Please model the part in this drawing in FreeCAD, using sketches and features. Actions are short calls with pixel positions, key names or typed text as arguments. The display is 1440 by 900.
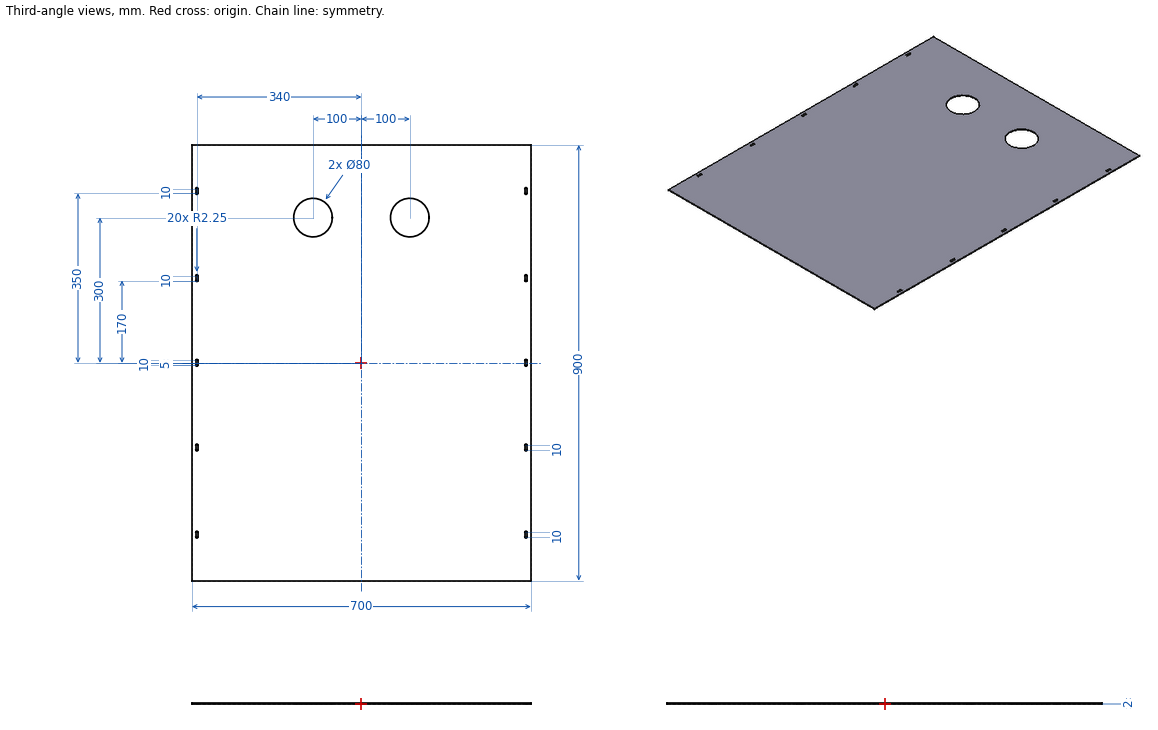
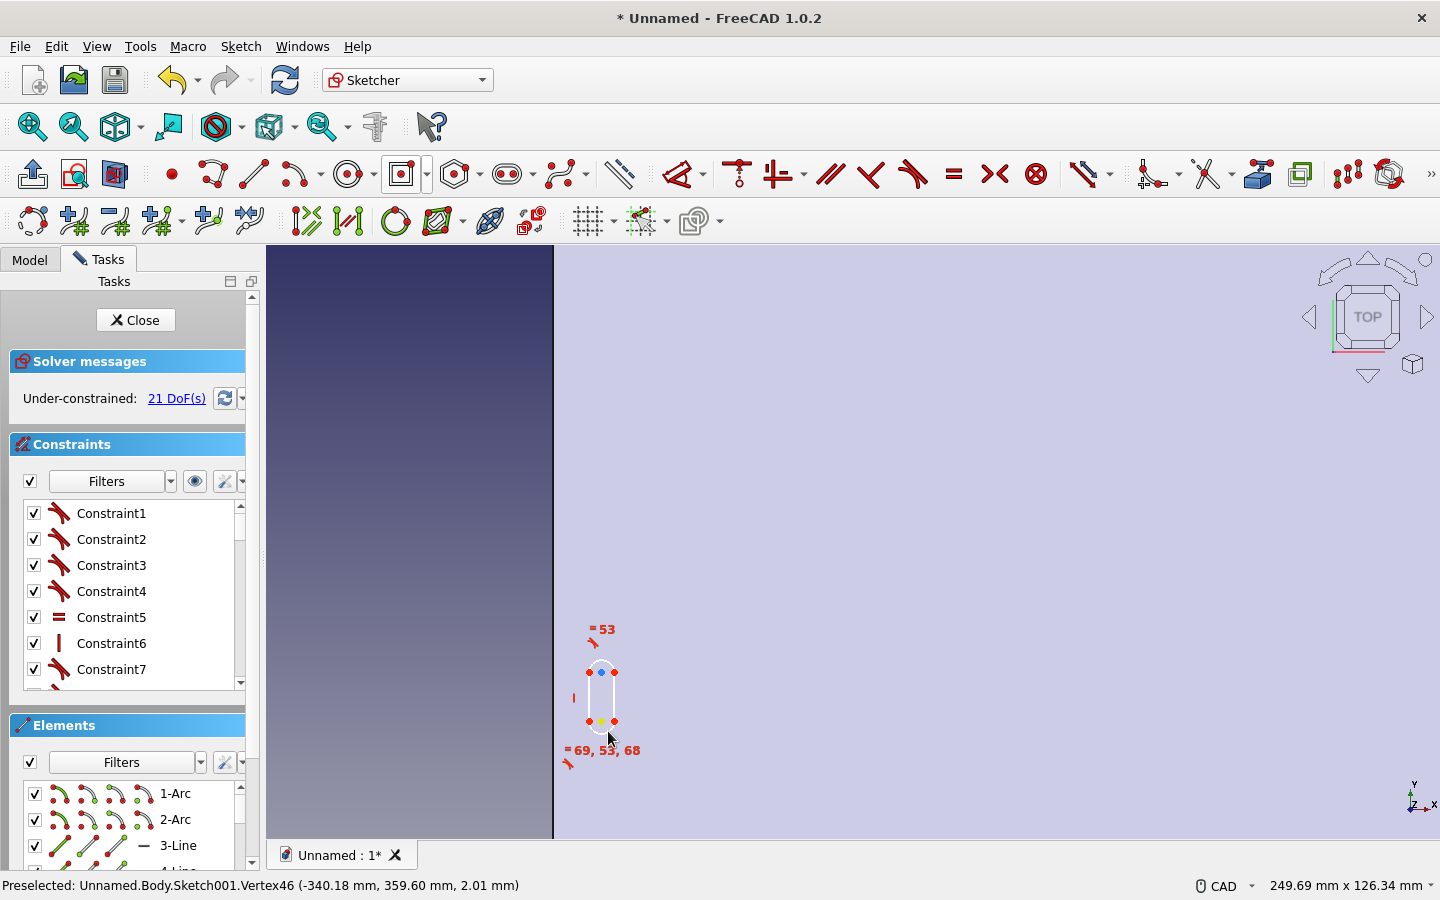
click(602, 721)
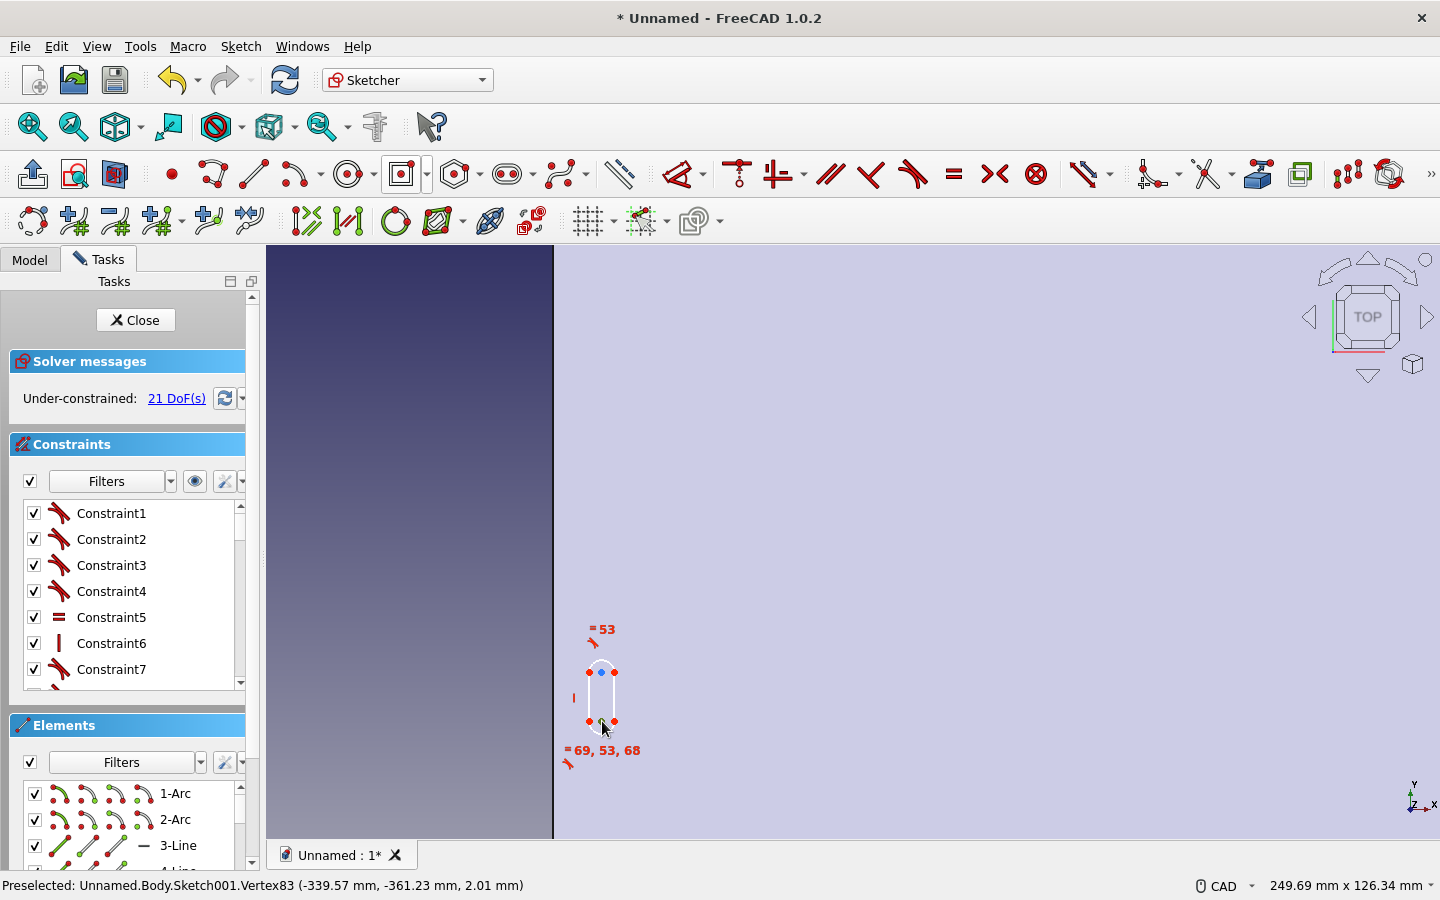
scroll(608, 731, down, 11)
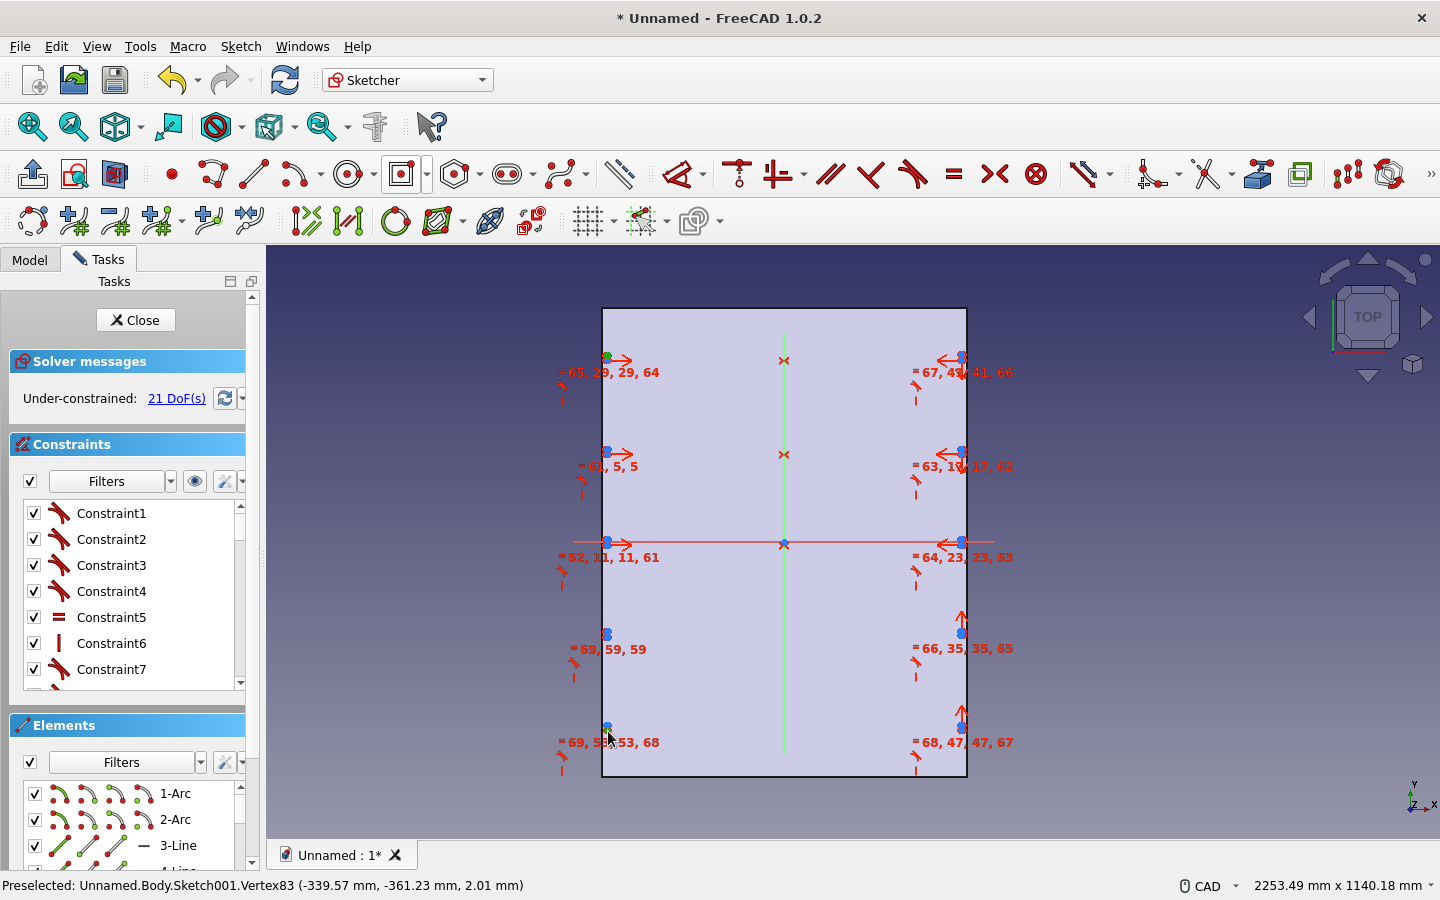
click(574, 542)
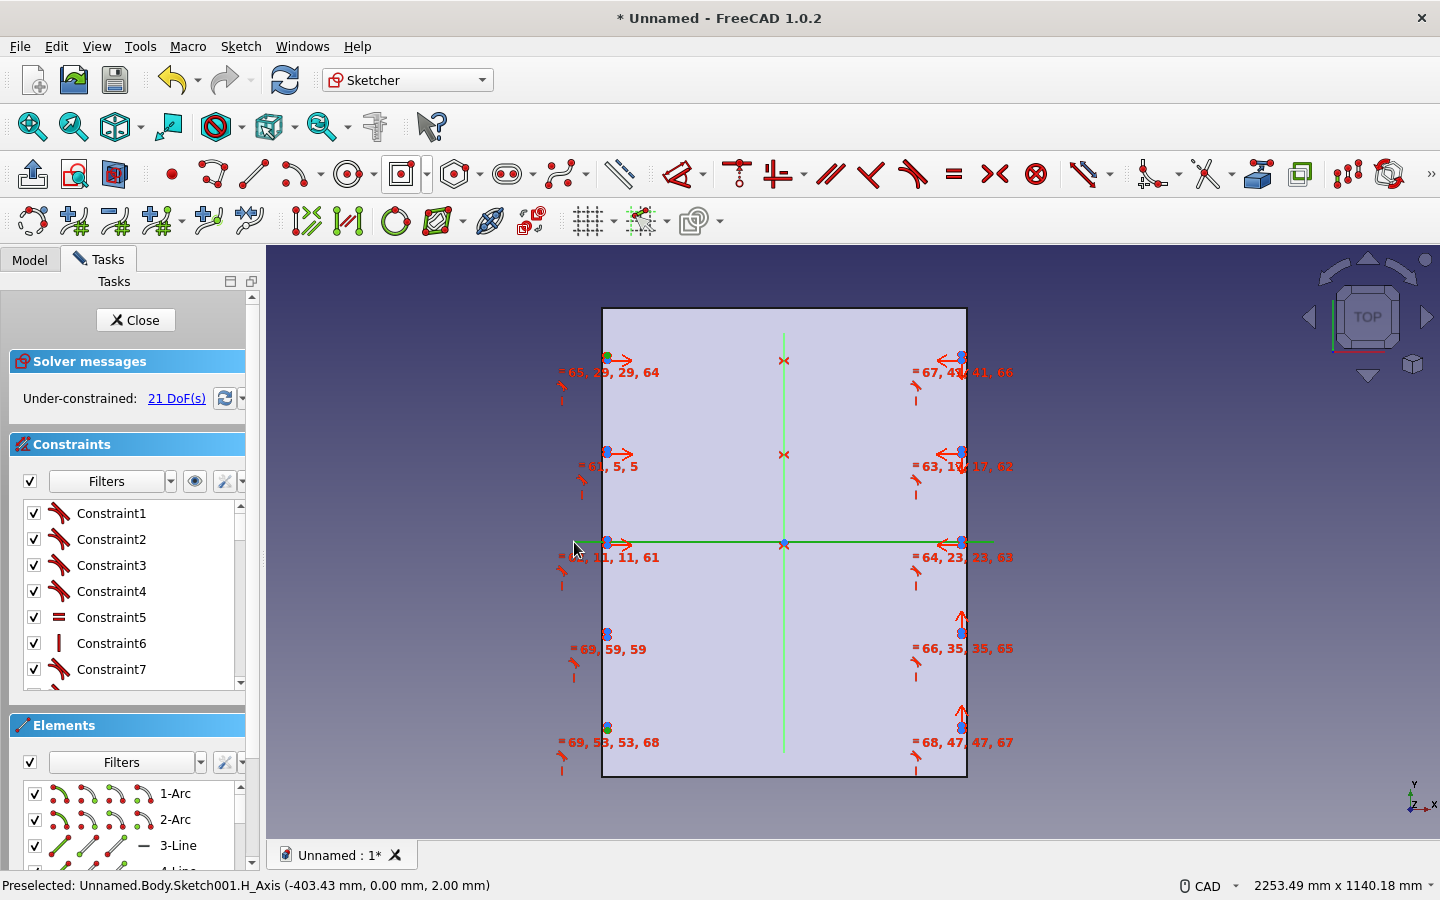
key(s)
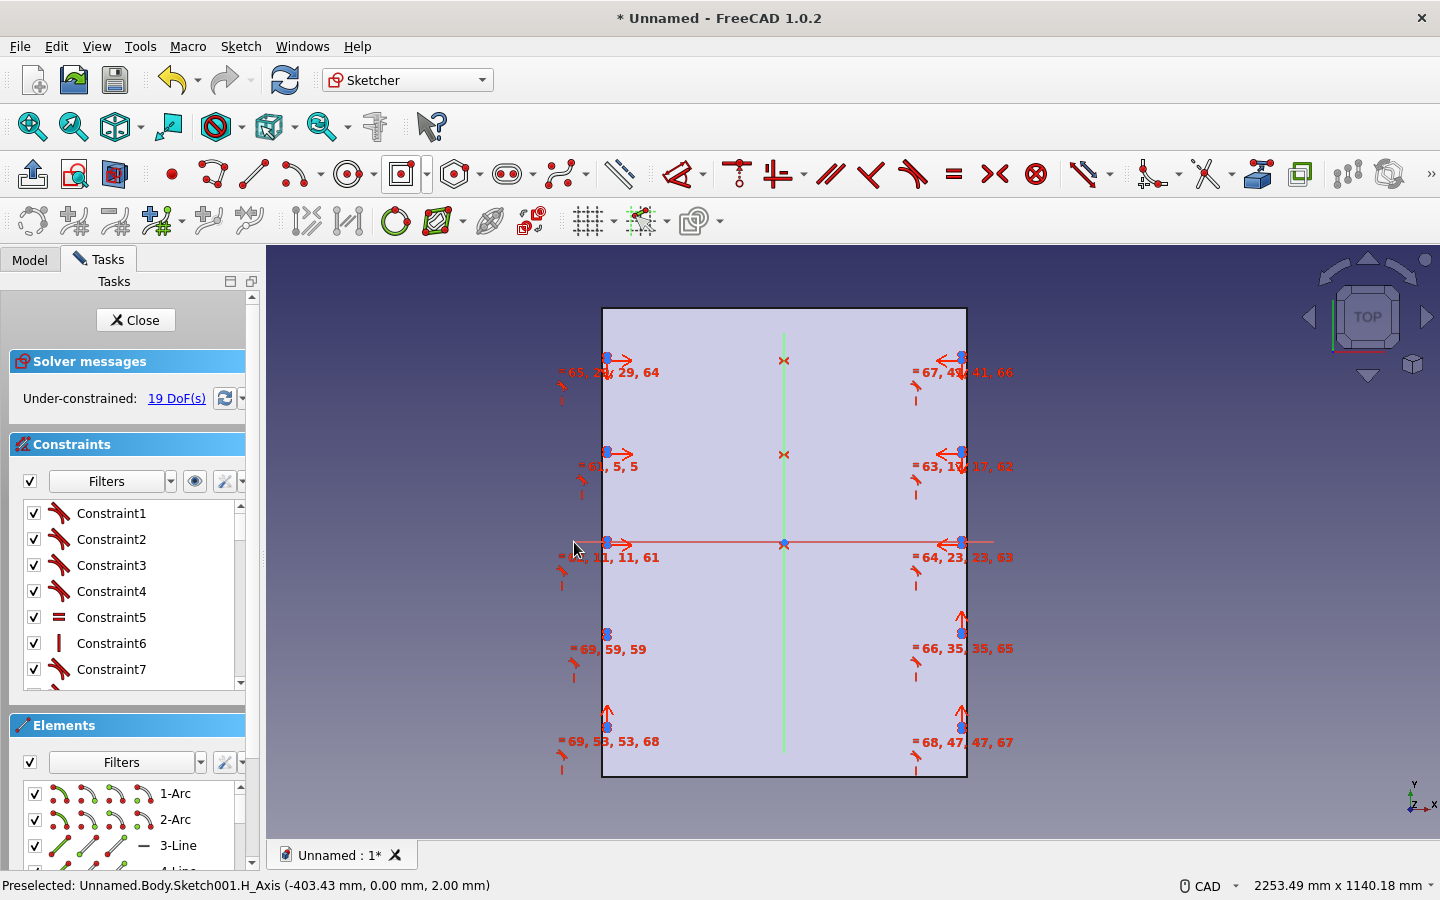
scroll(607, 449, up, 11)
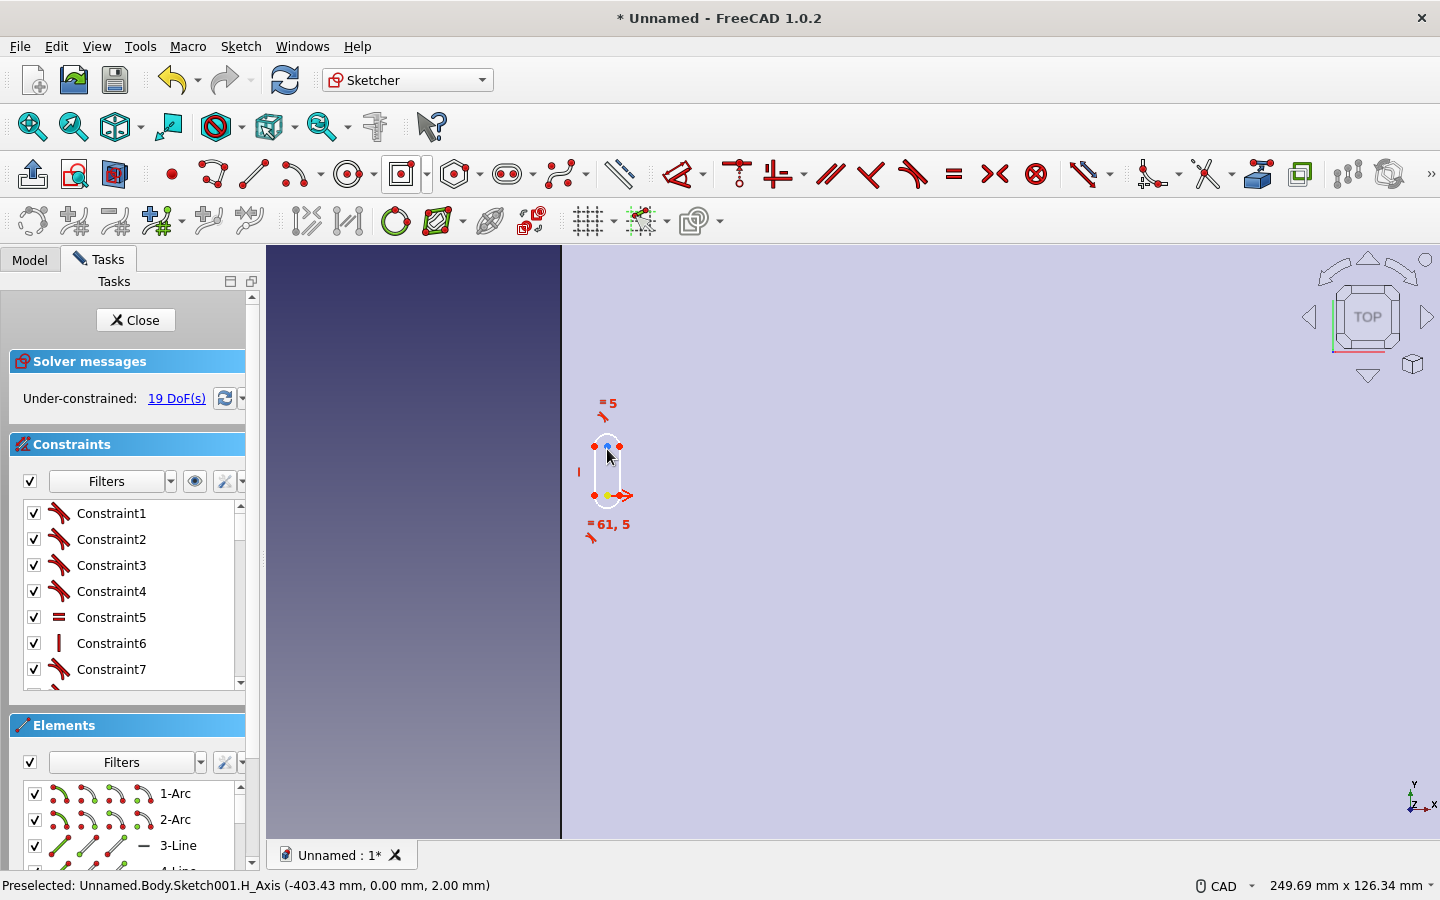
click(607, 447)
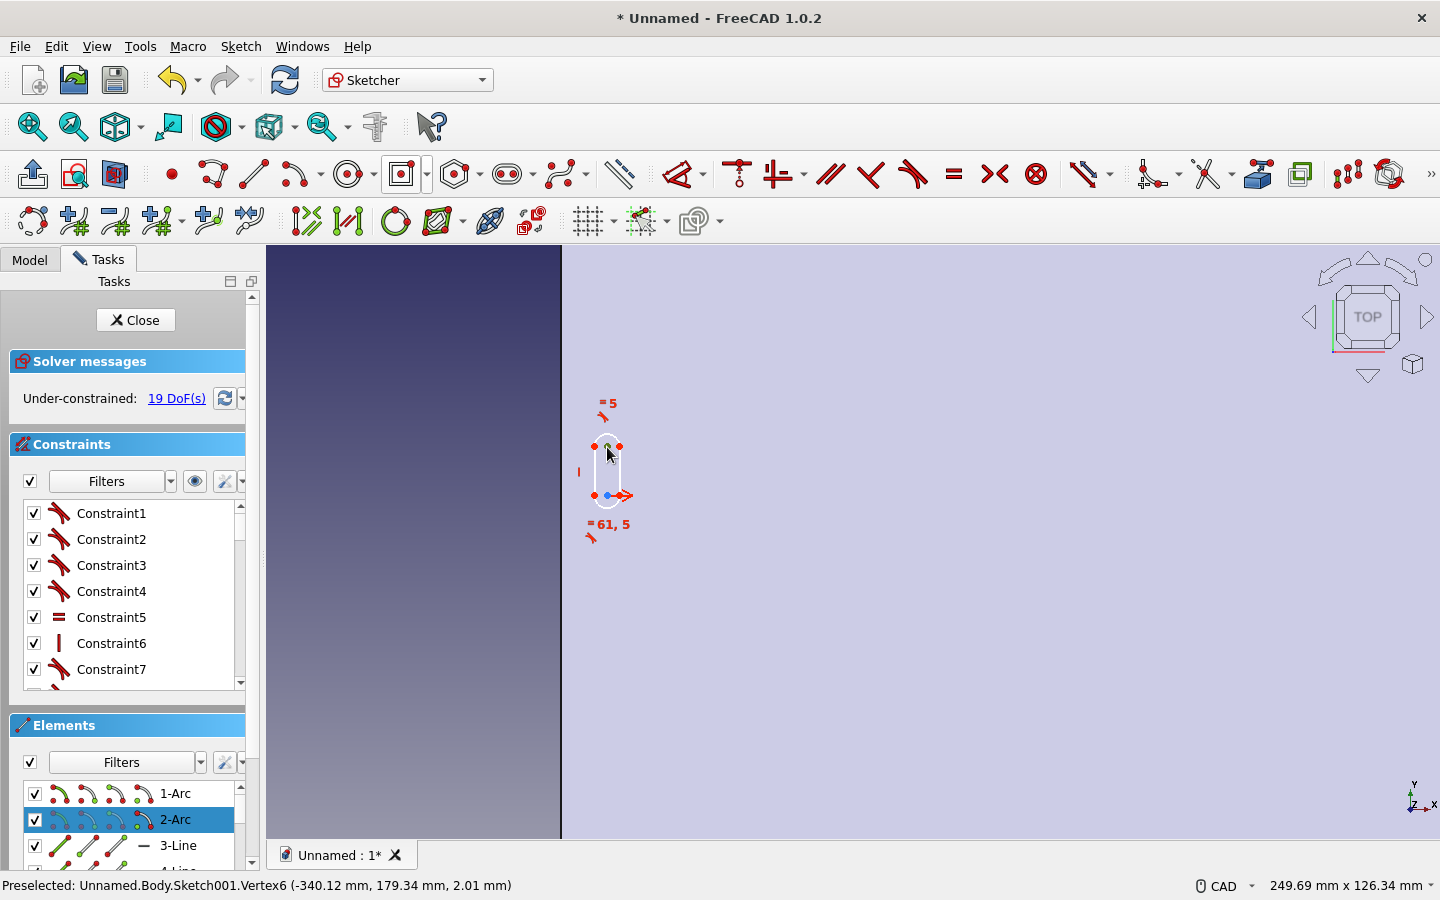
scroll(607, 449, down, 11)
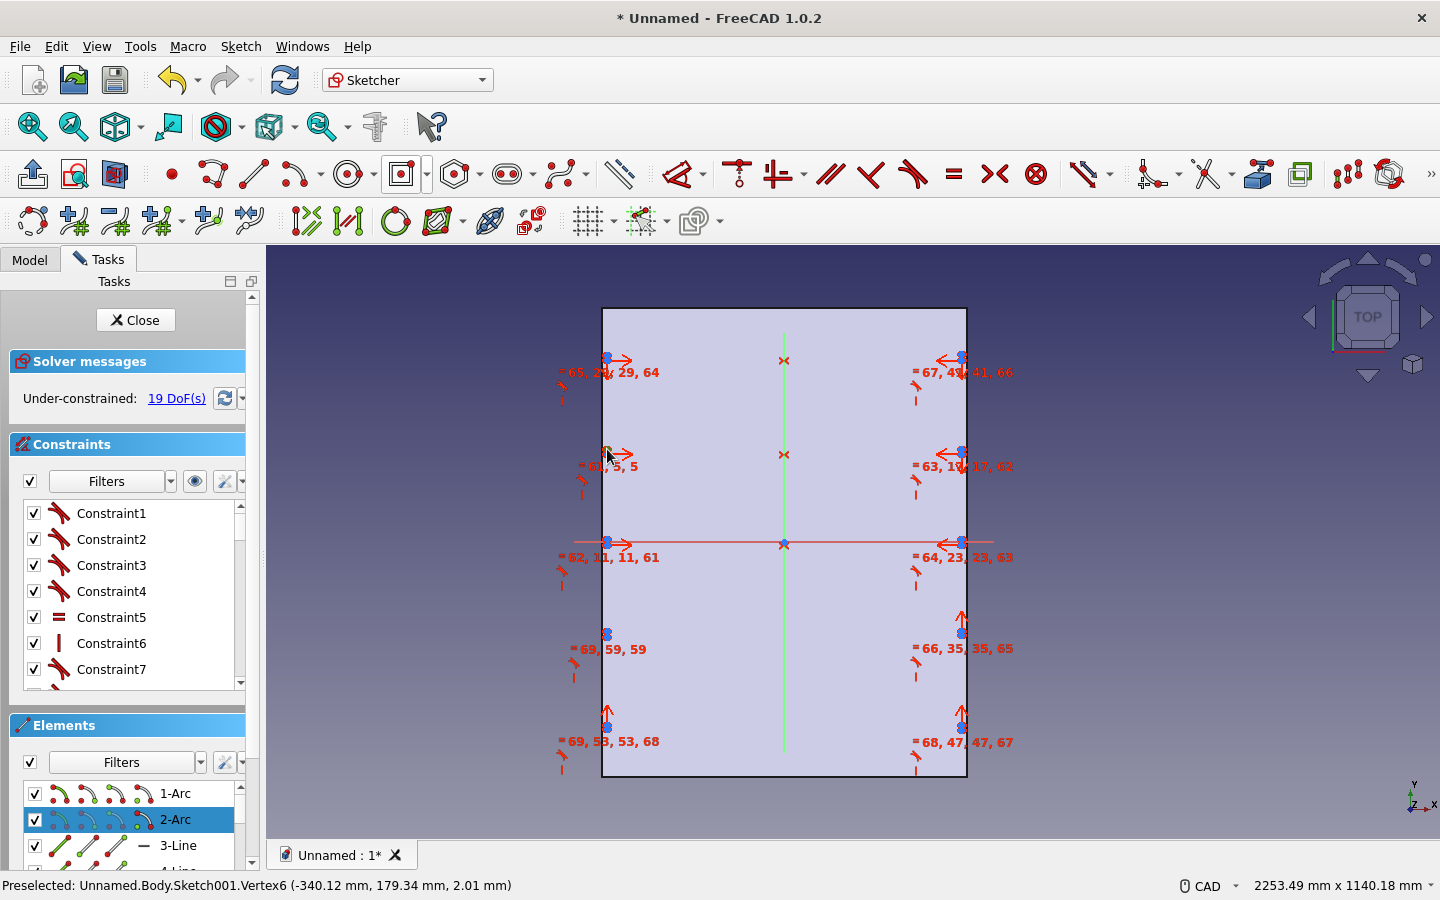
scroll(607, 637, up, 11)